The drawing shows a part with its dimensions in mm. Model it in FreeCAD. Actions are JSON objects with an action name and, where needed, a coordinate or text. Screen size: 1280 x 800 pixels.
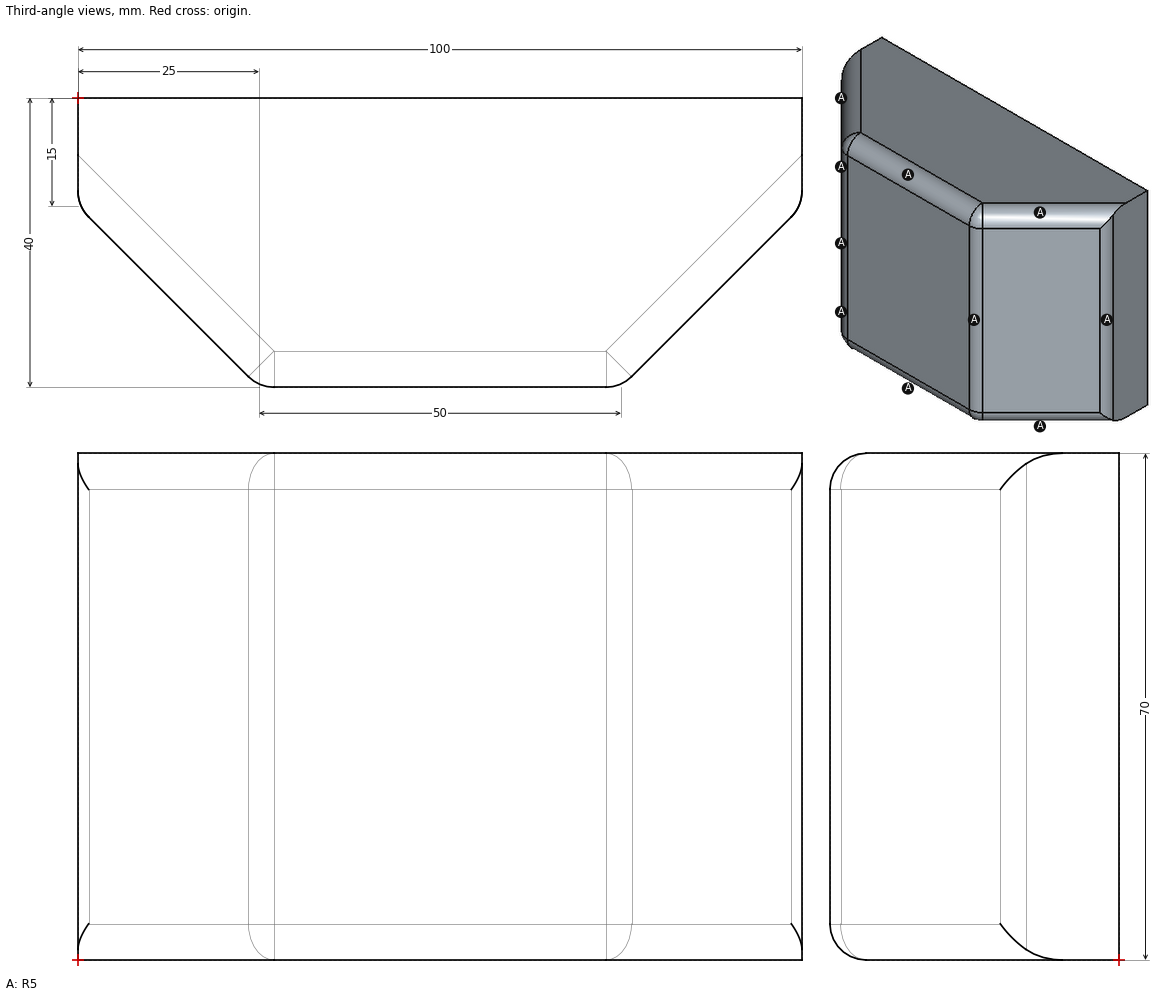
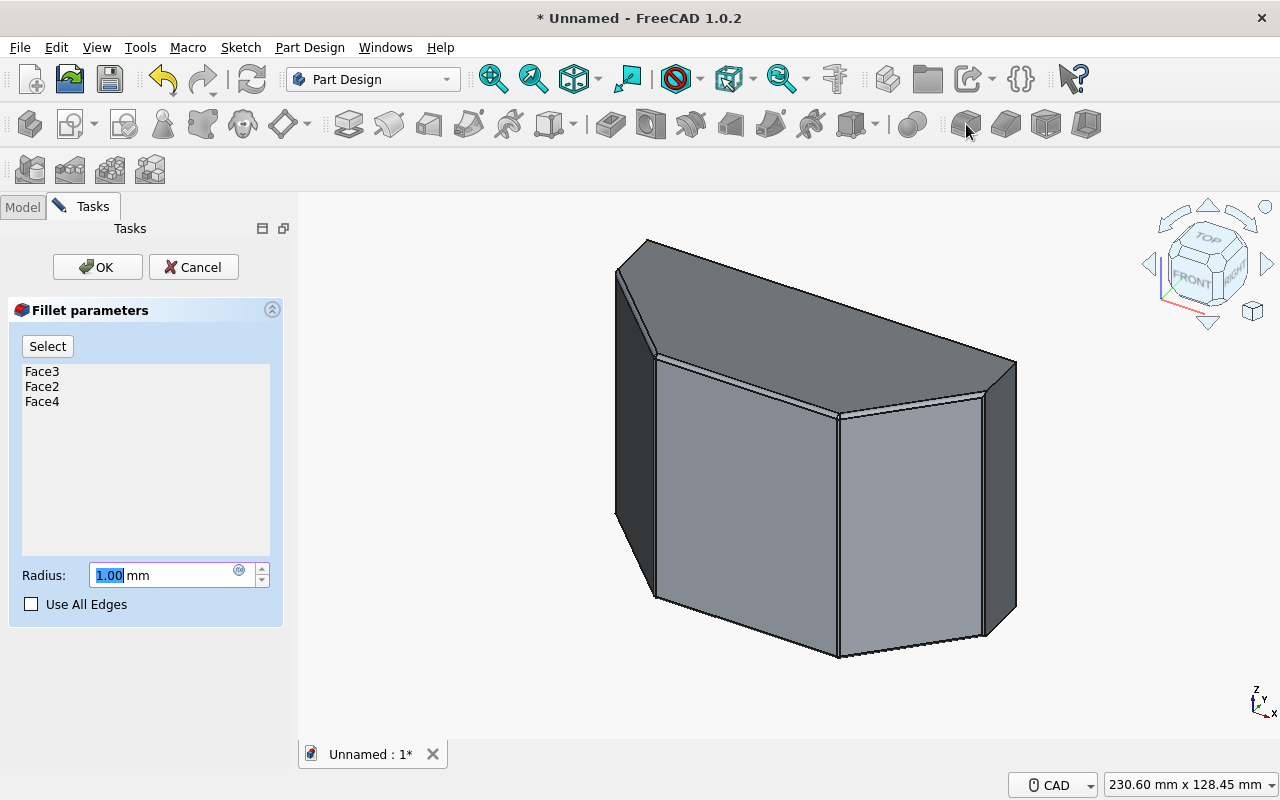
{"action": "type", "text": "5"}
{"action": "key", "text": "Tab"}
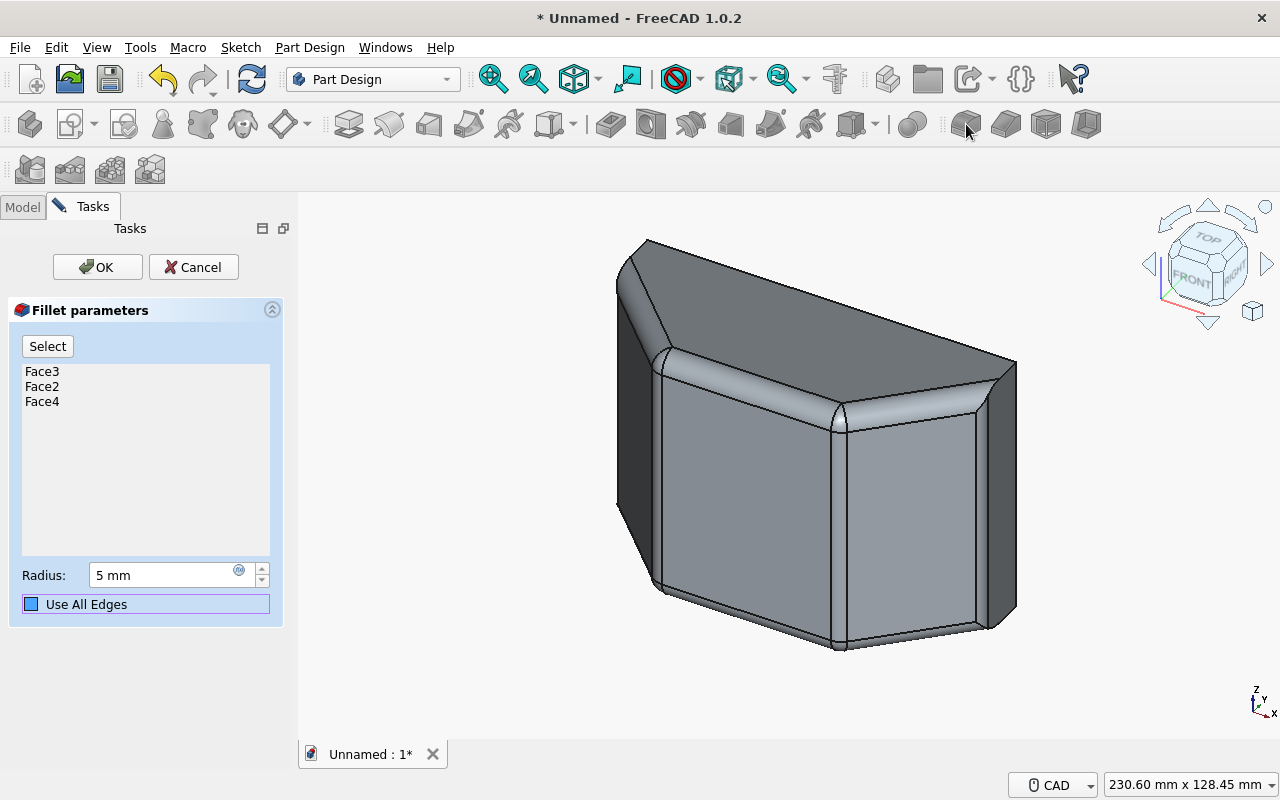
{"action": "left_click", "coordinate": [98, 267]}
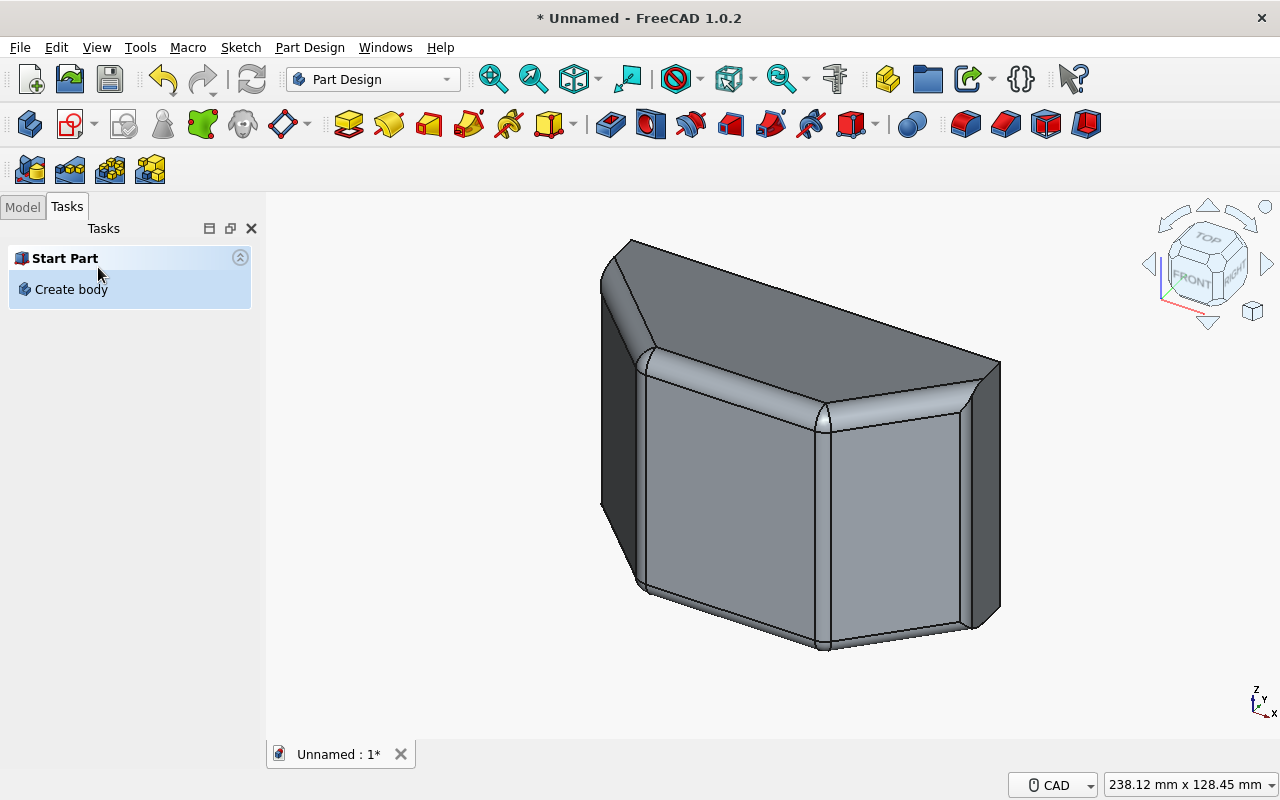
{"action": "key", "text": "0"}